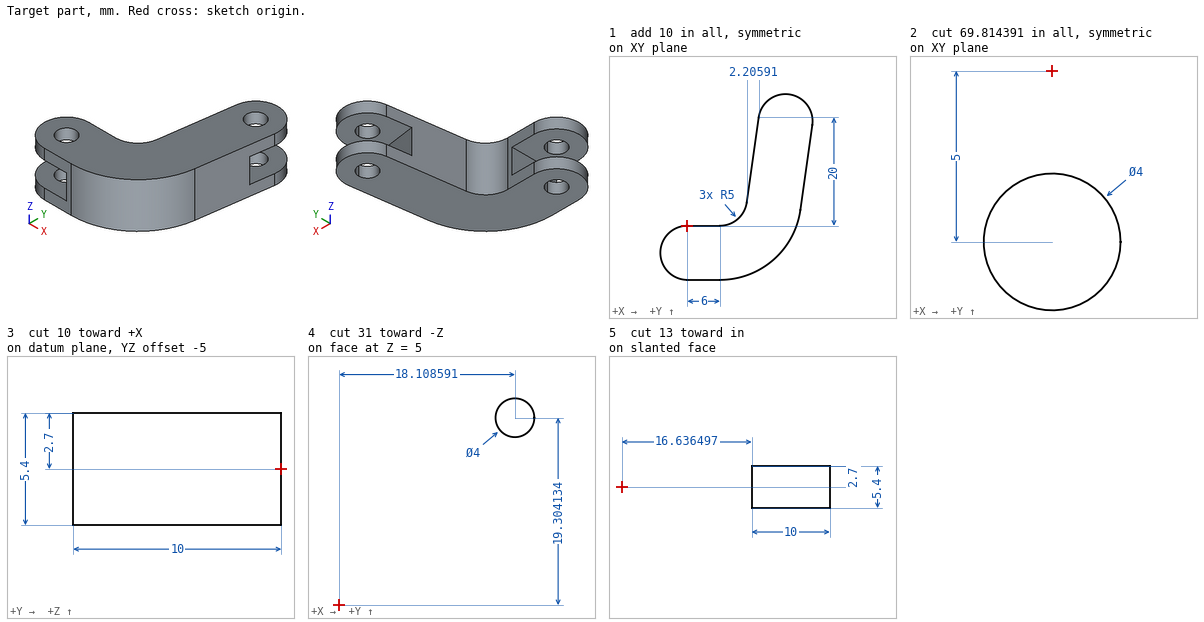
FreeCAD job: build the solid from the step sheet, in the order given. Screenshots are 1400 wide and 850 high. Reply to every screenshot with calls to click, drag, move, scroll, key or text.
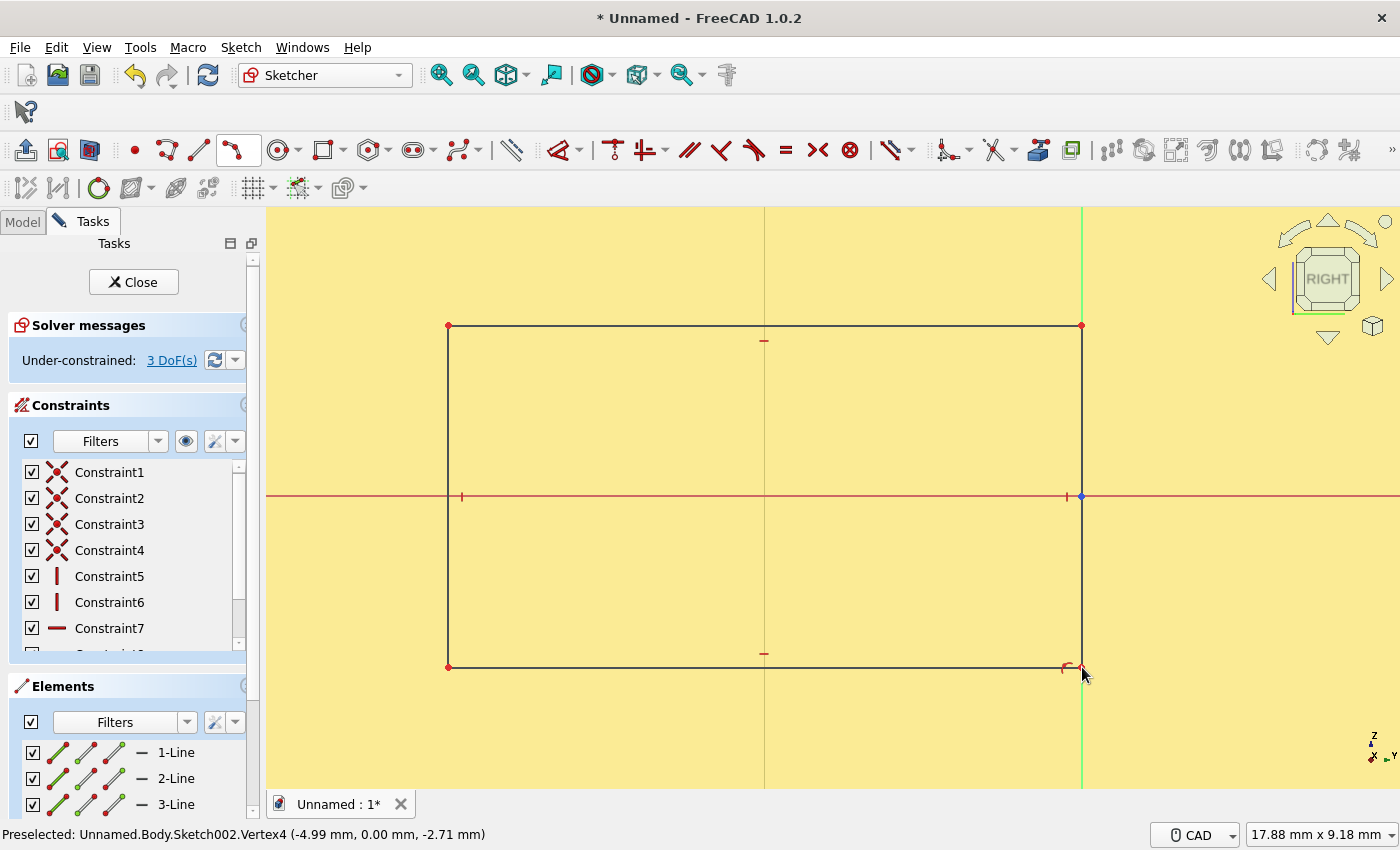
click(558, 150)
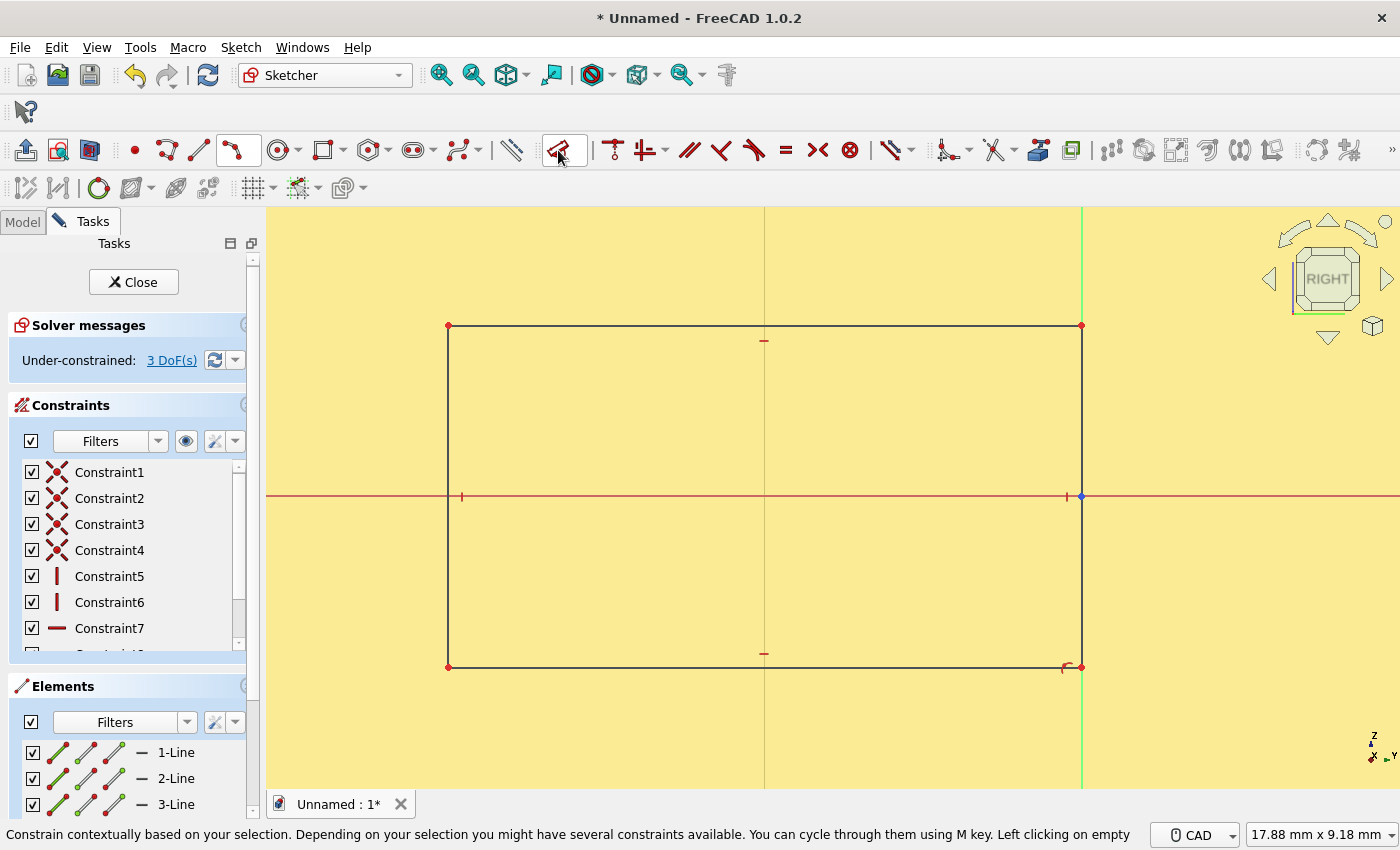
click(638, 668)
click(765, 702)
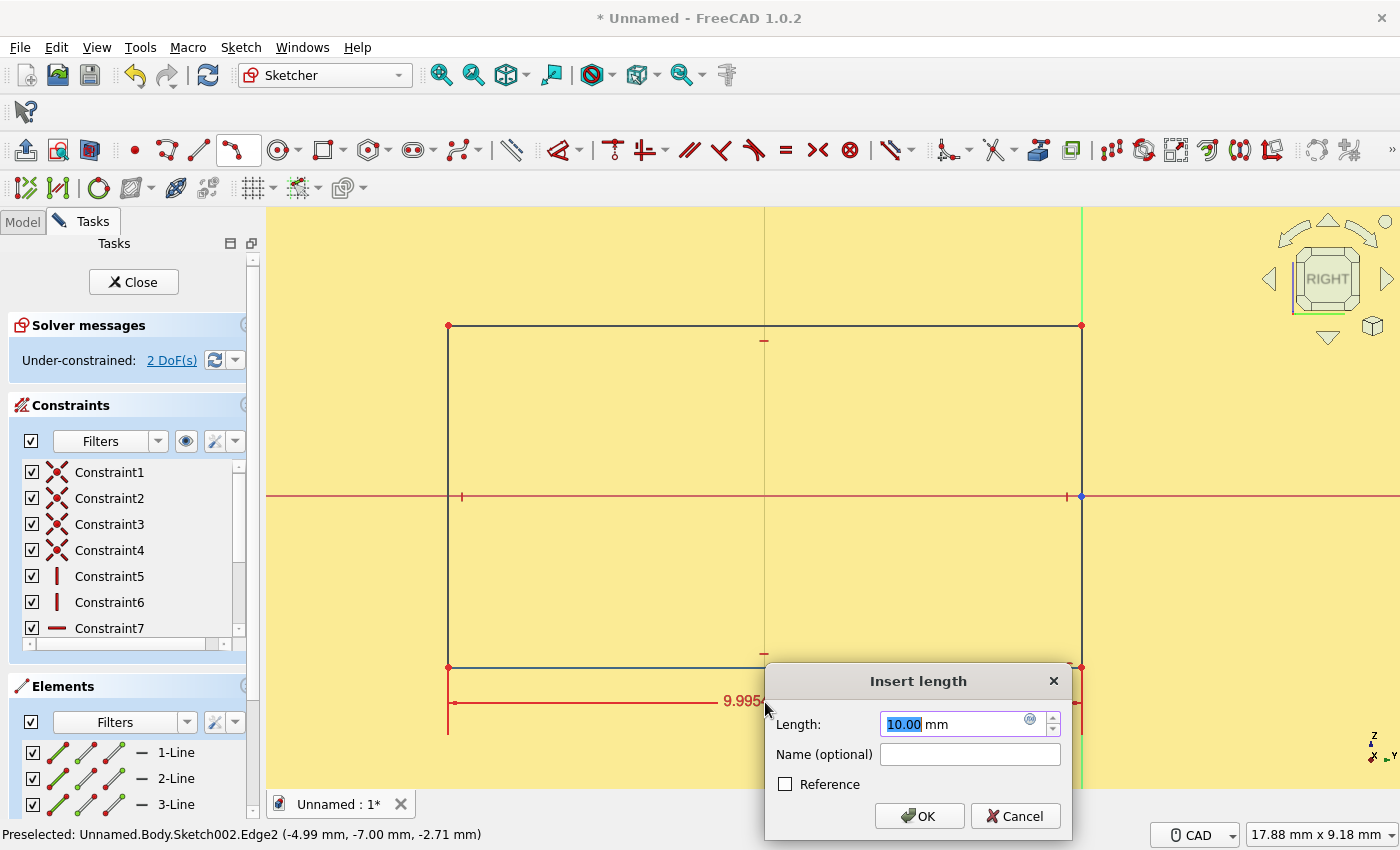
text(10)
key(Return)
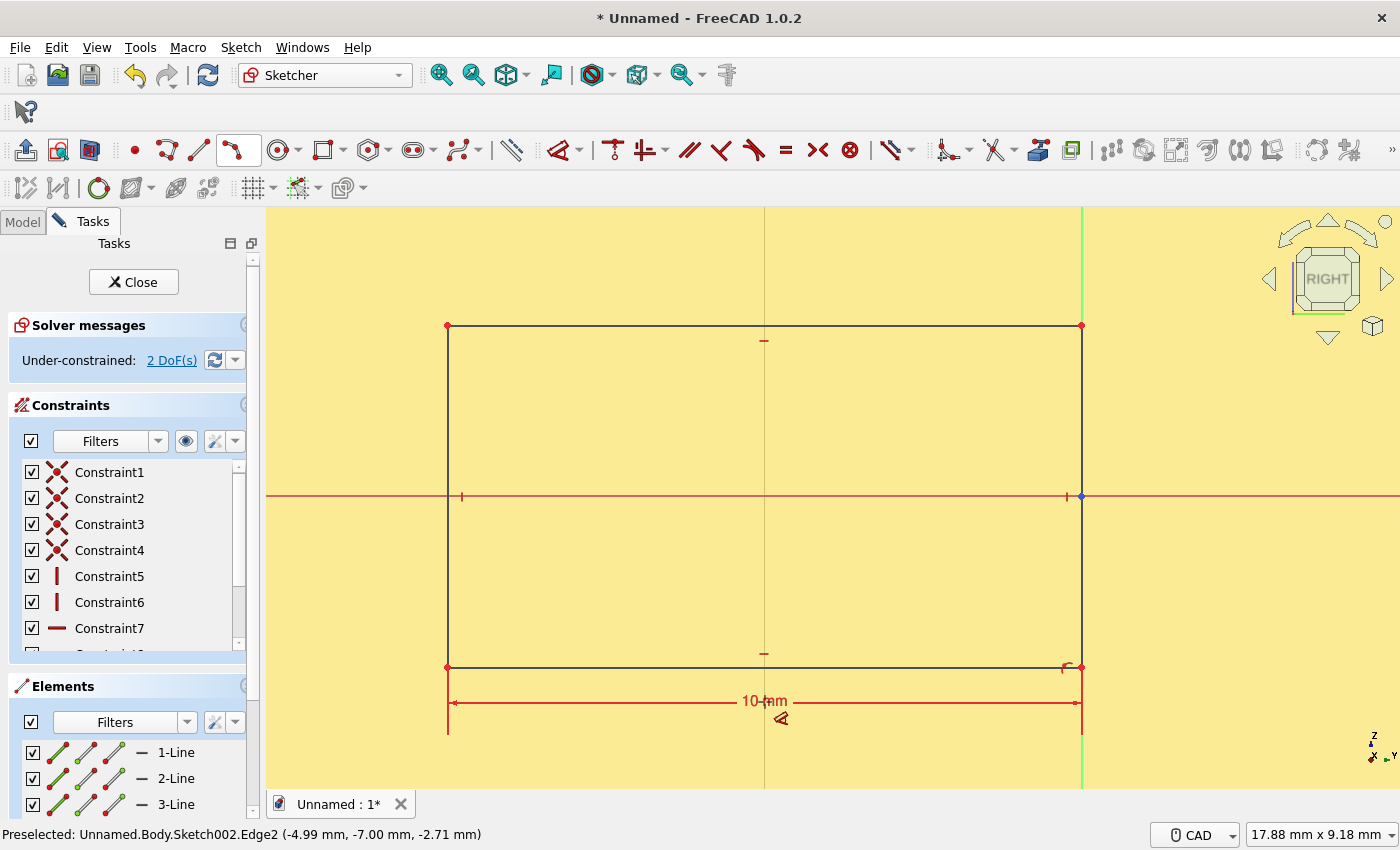
click(448, 429)
click(414, 418)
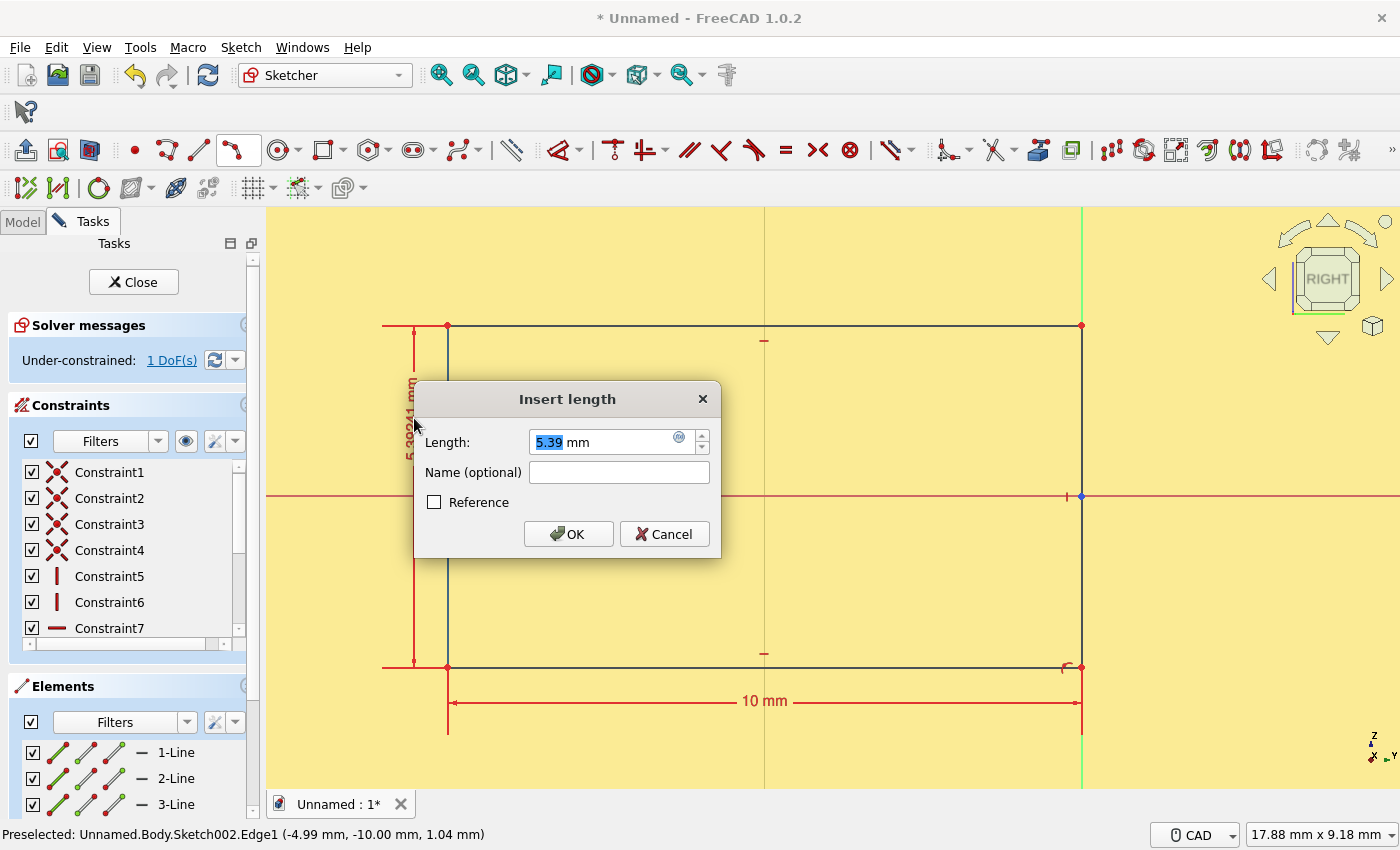
text(5.4)
key(Return)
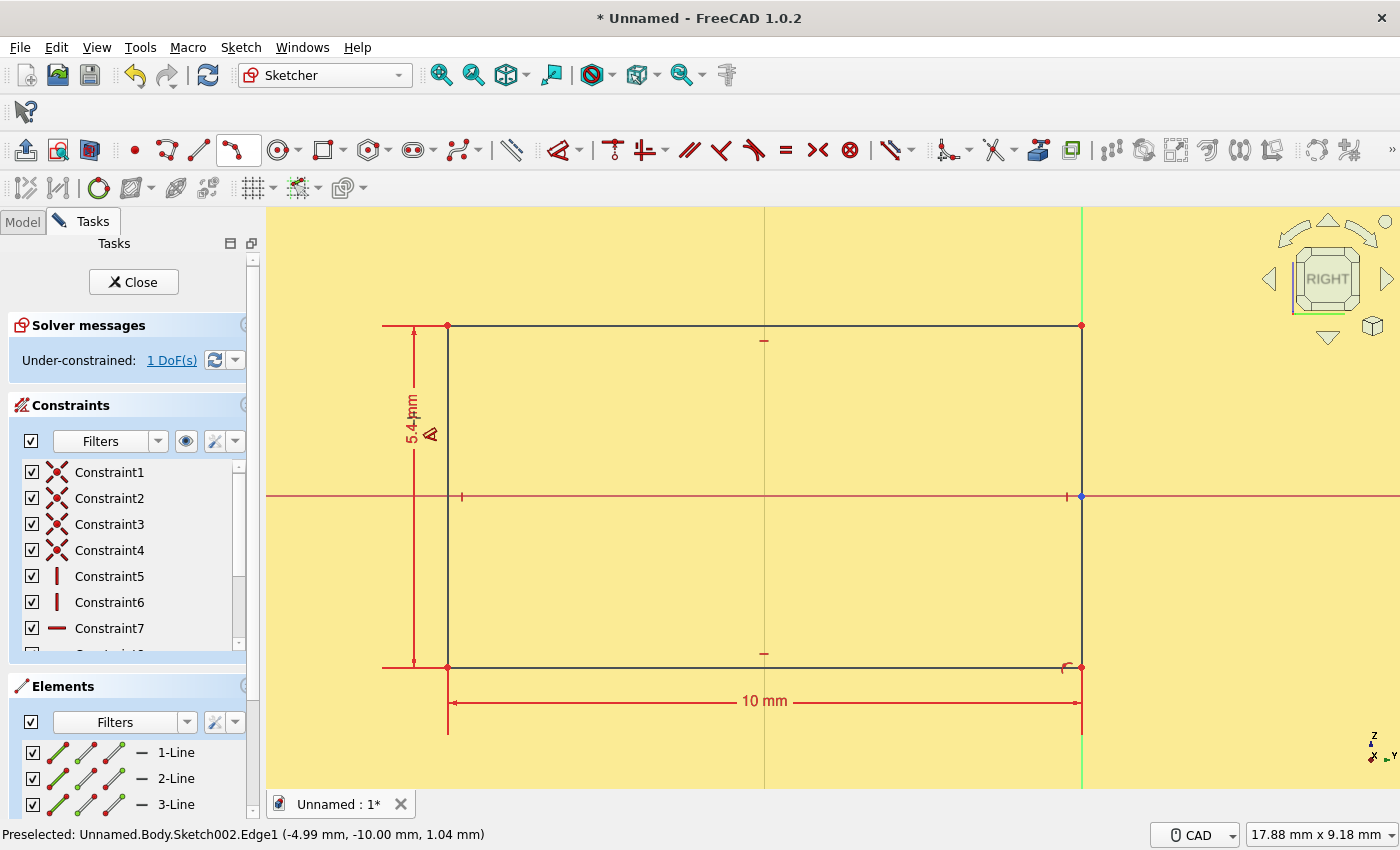
click(448, 326)
click(1116, 411)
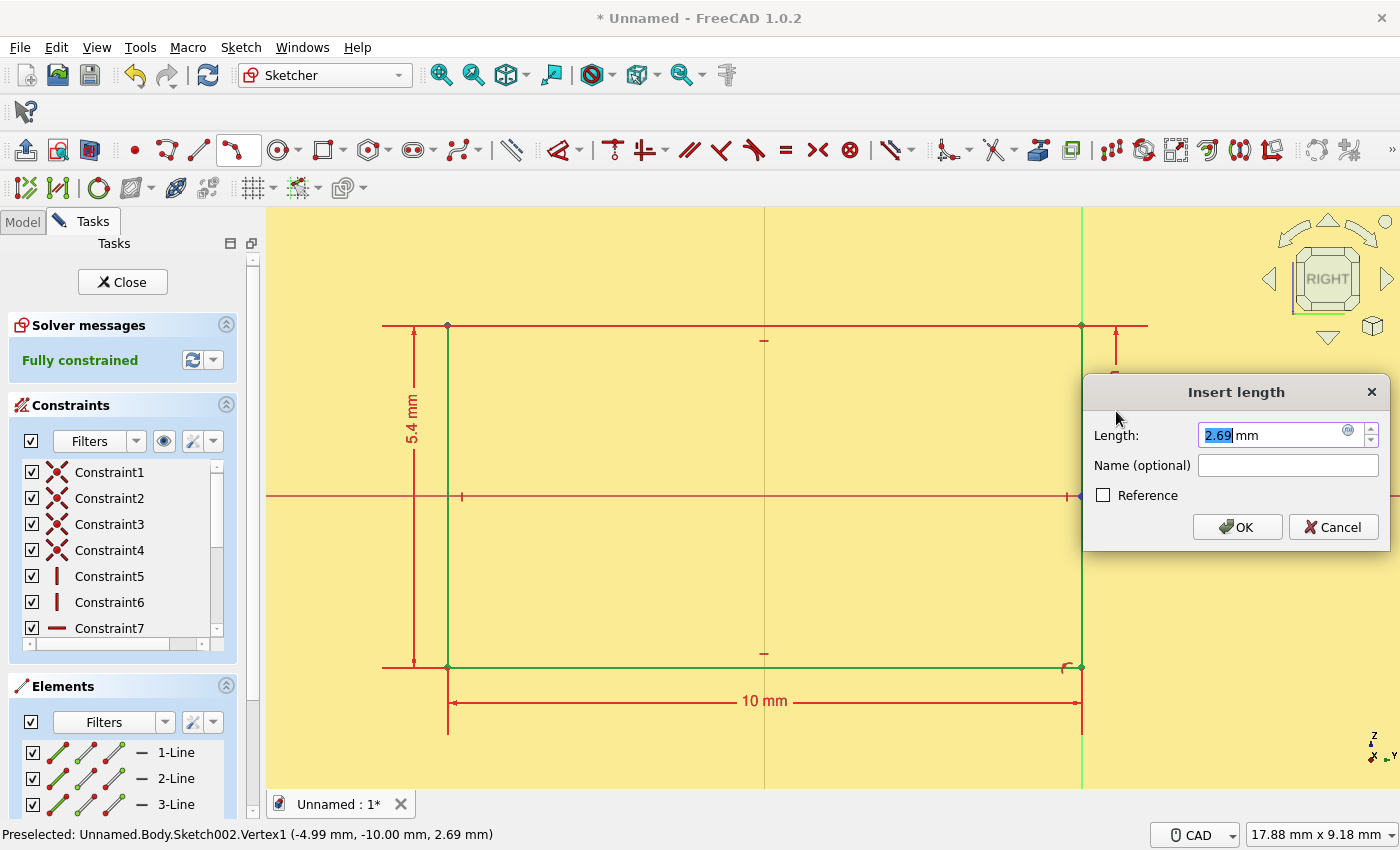
text(2.7)
key(Return)
key(Escape)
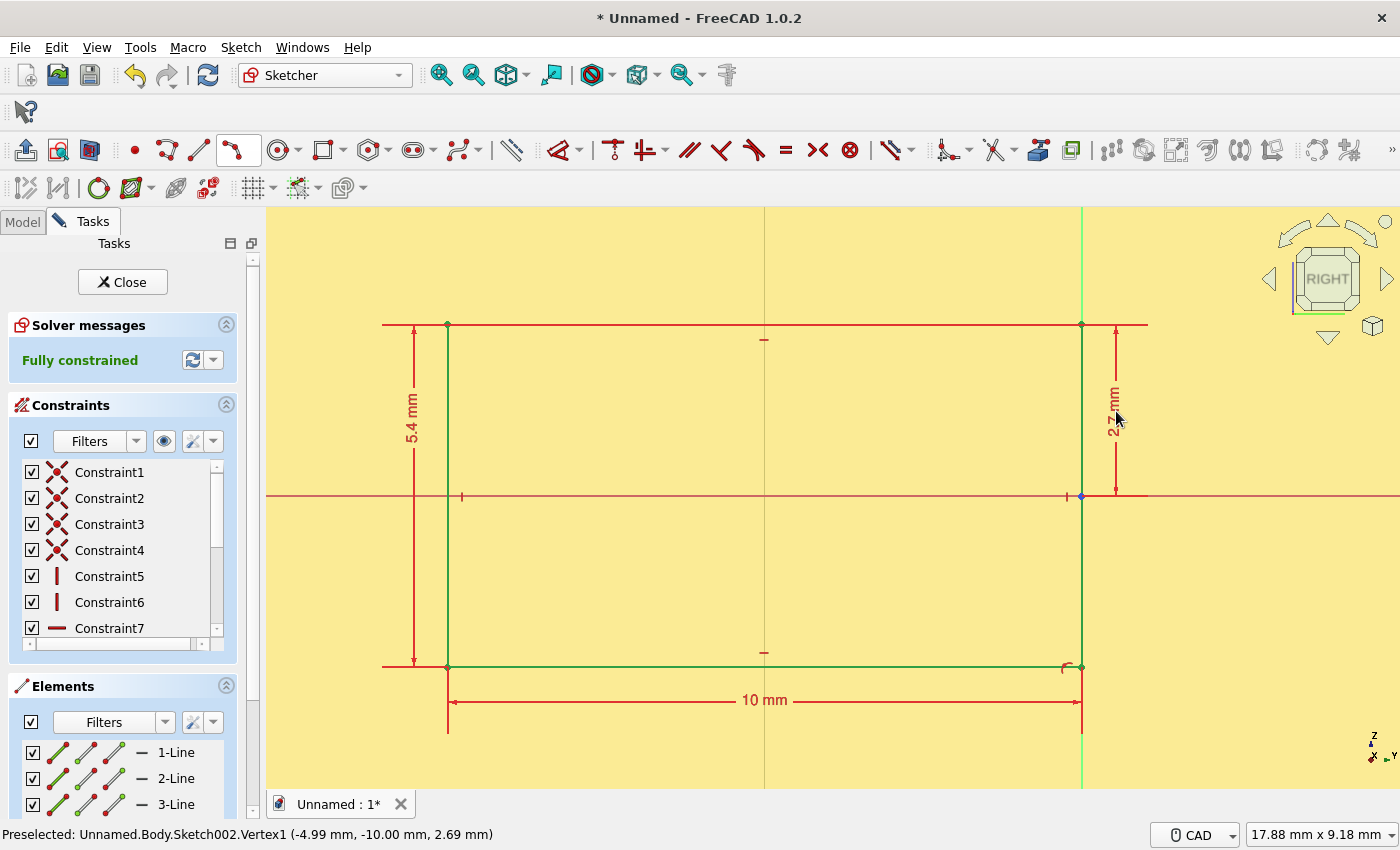
click(123, 282)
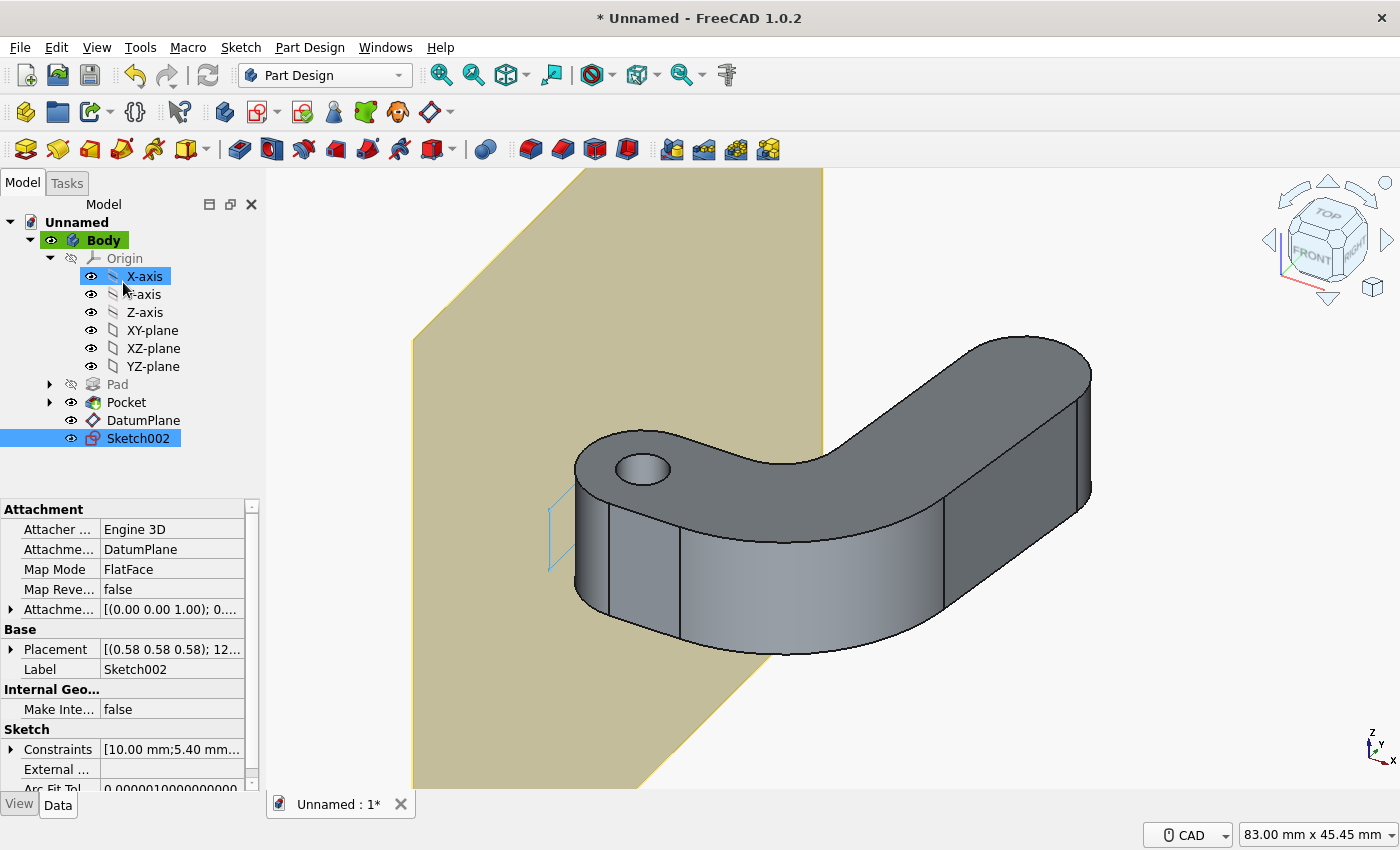
click(240, 150)